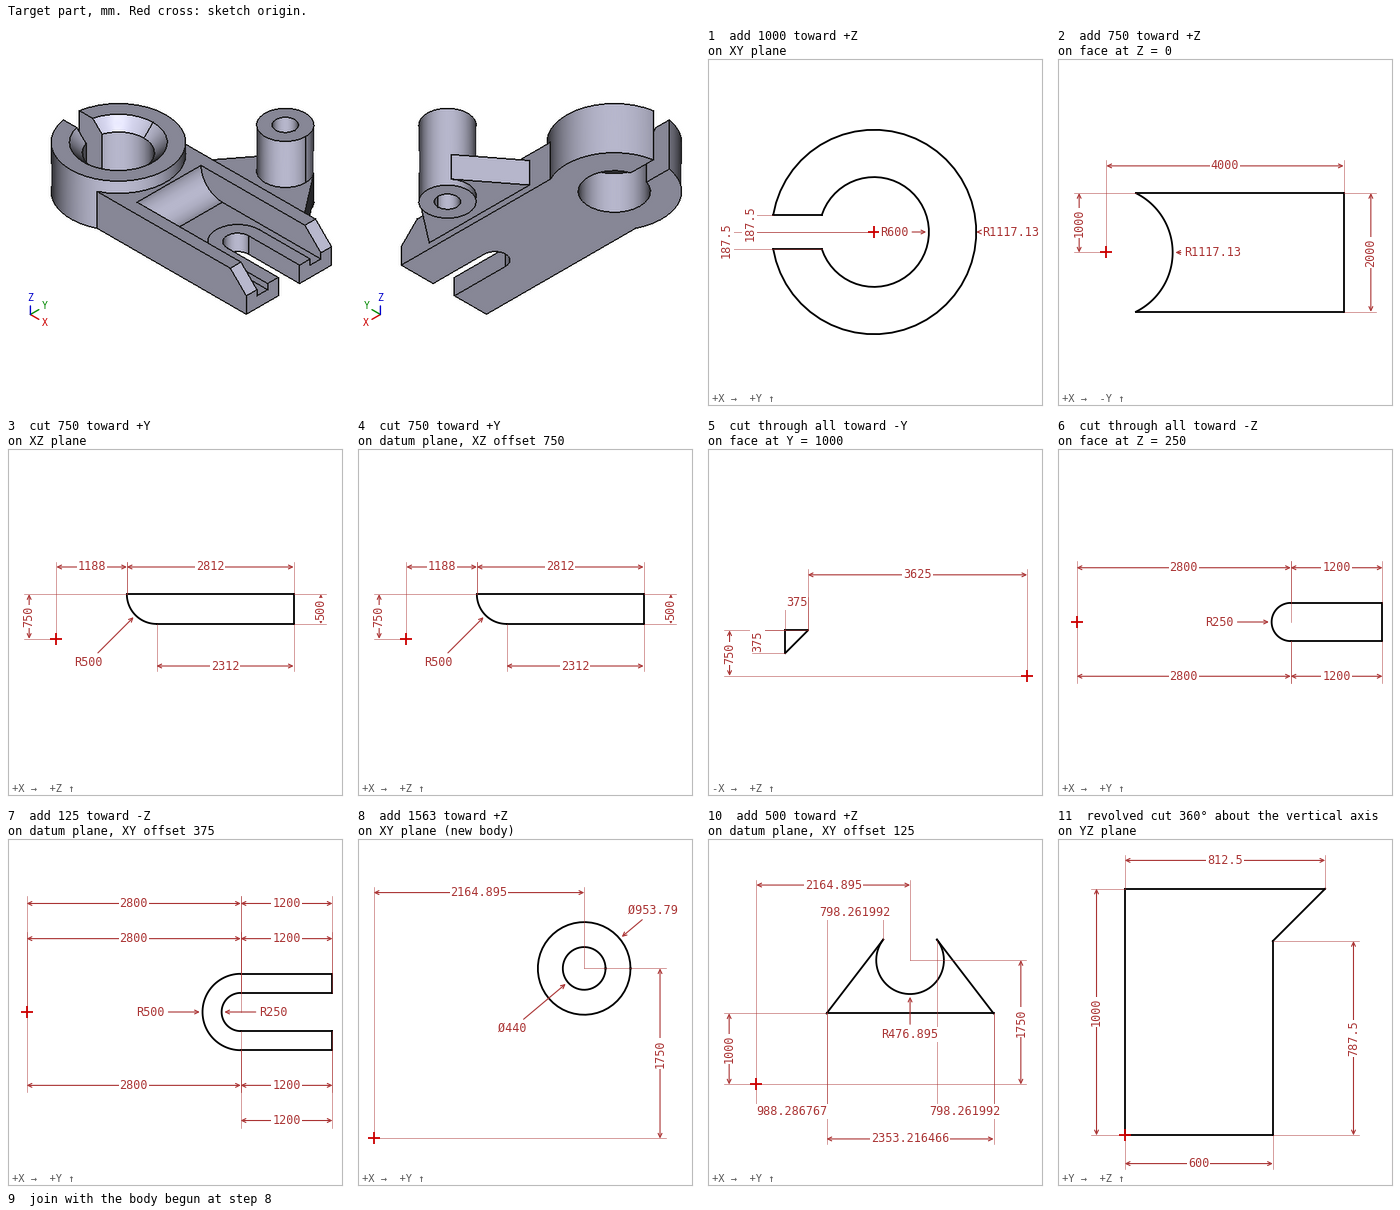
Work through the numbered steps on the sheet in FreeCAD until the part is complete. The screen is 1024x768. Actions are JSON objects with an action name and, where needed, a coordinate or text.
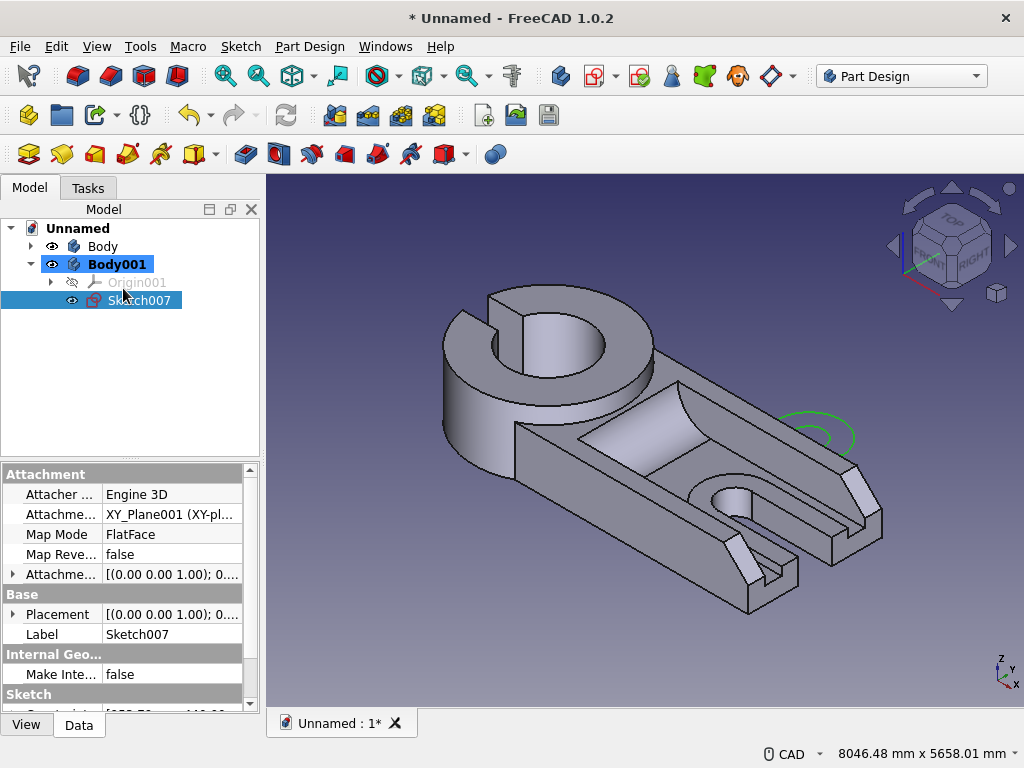
{"action": "left_click", "coordinate": [29, 154]}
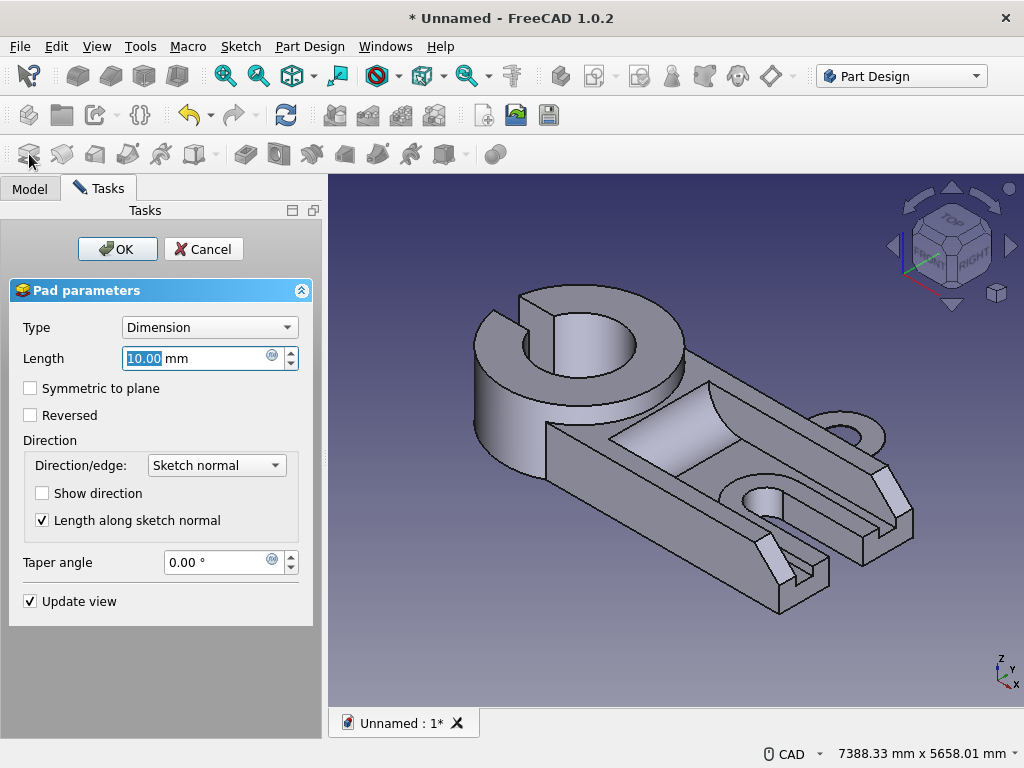
{"action": "type", "text": "1563"}
{"action": "key", "text": "Tab"}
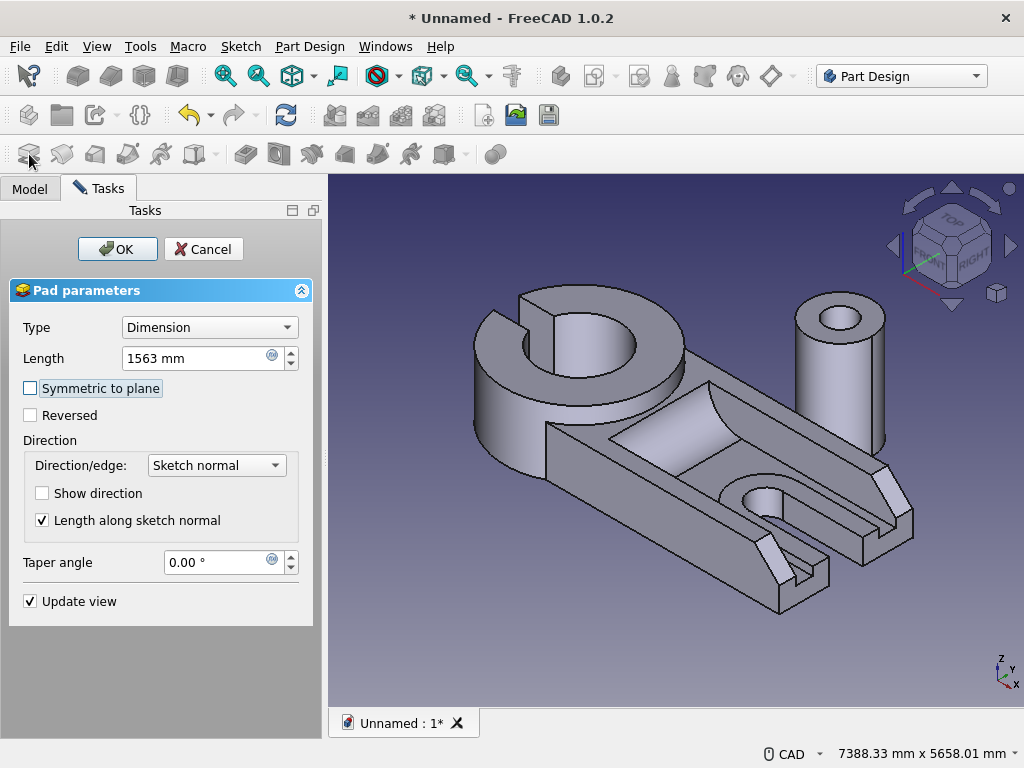
{"action": "left_click", "coordinate": [118, 249]}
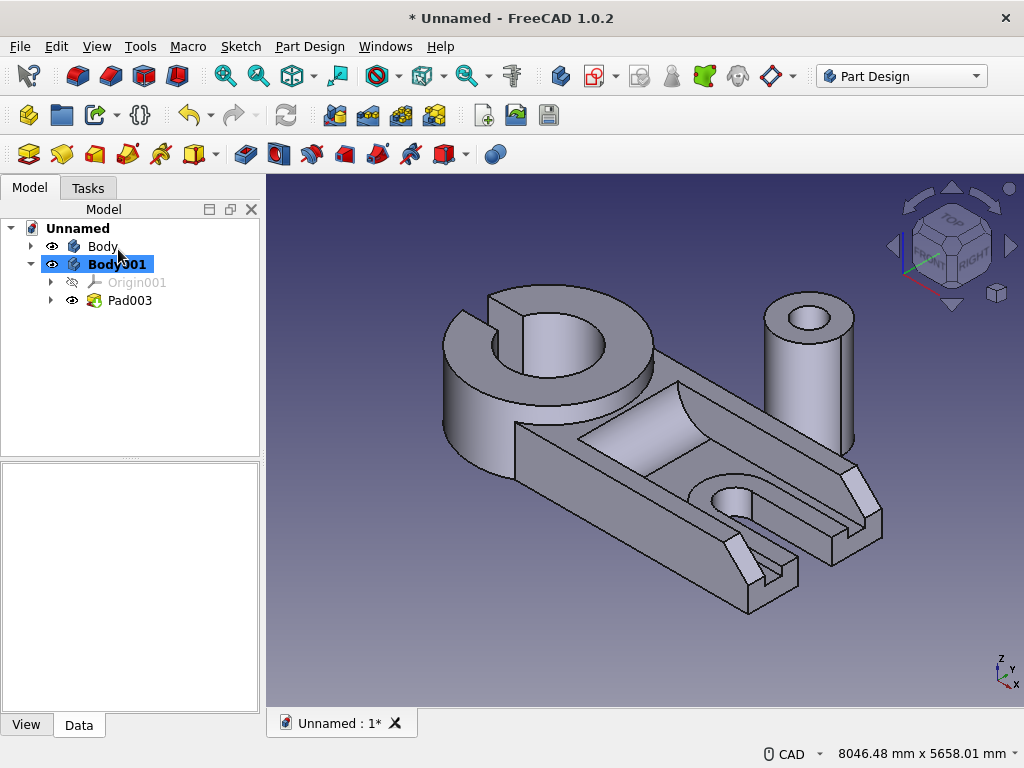
{"action": "key", "text": "v f"}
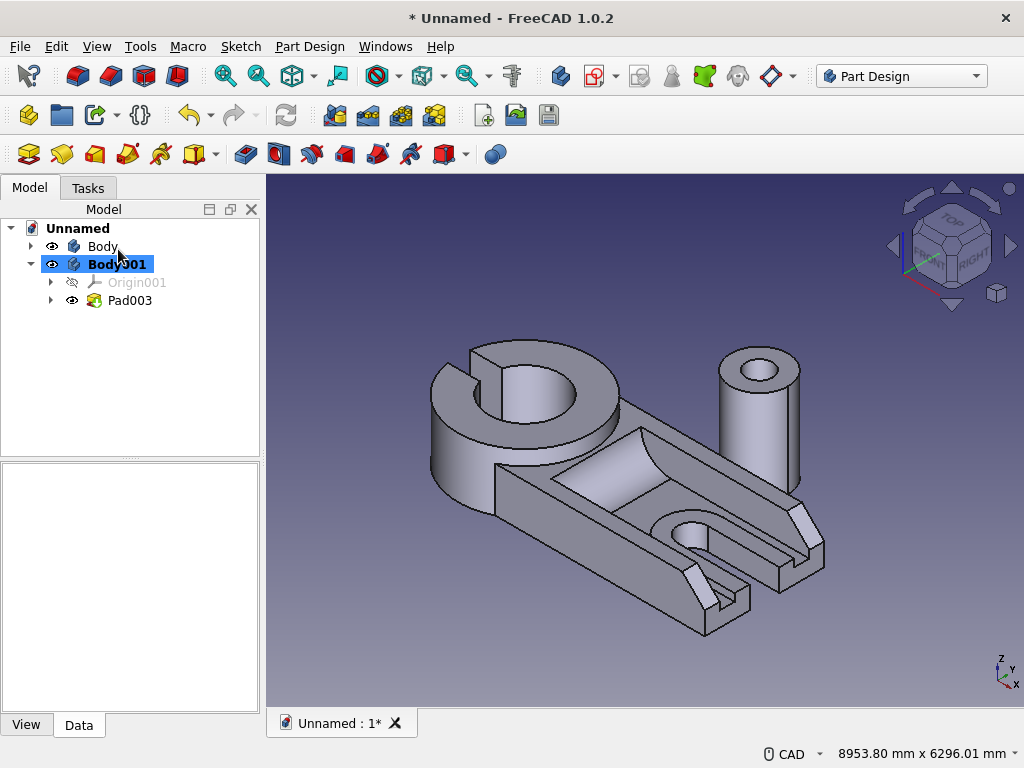
{"action": "double_click", "coordinate": [97, 246]}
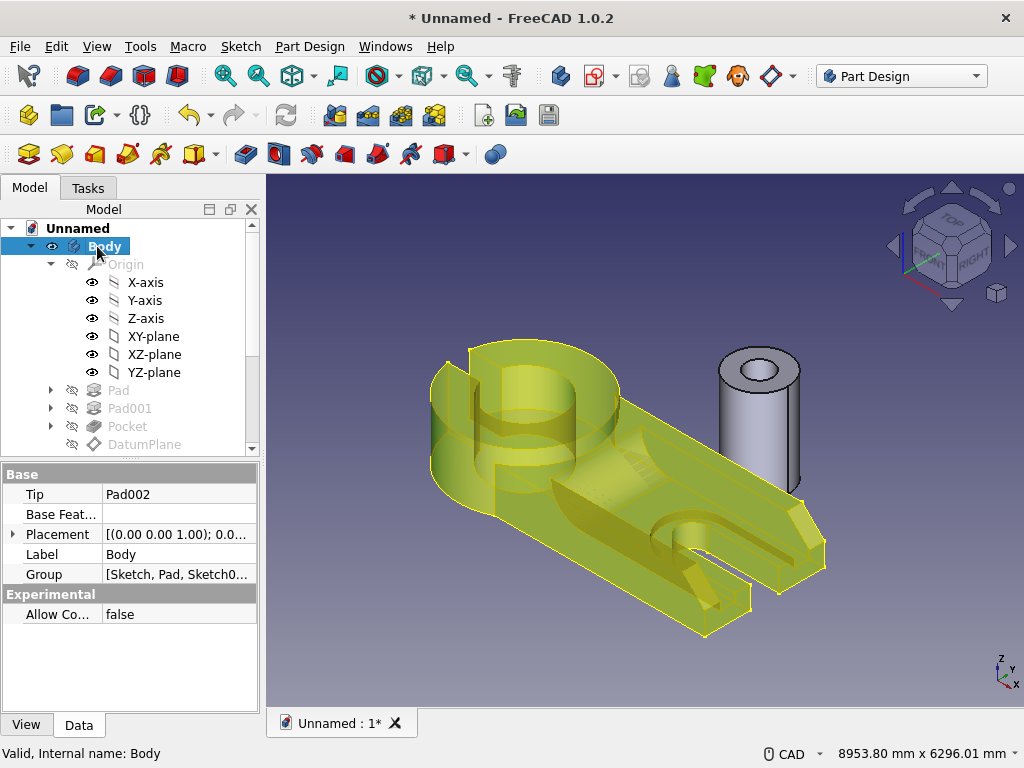
{"action": "left_click", "coordinate": [97, 246]}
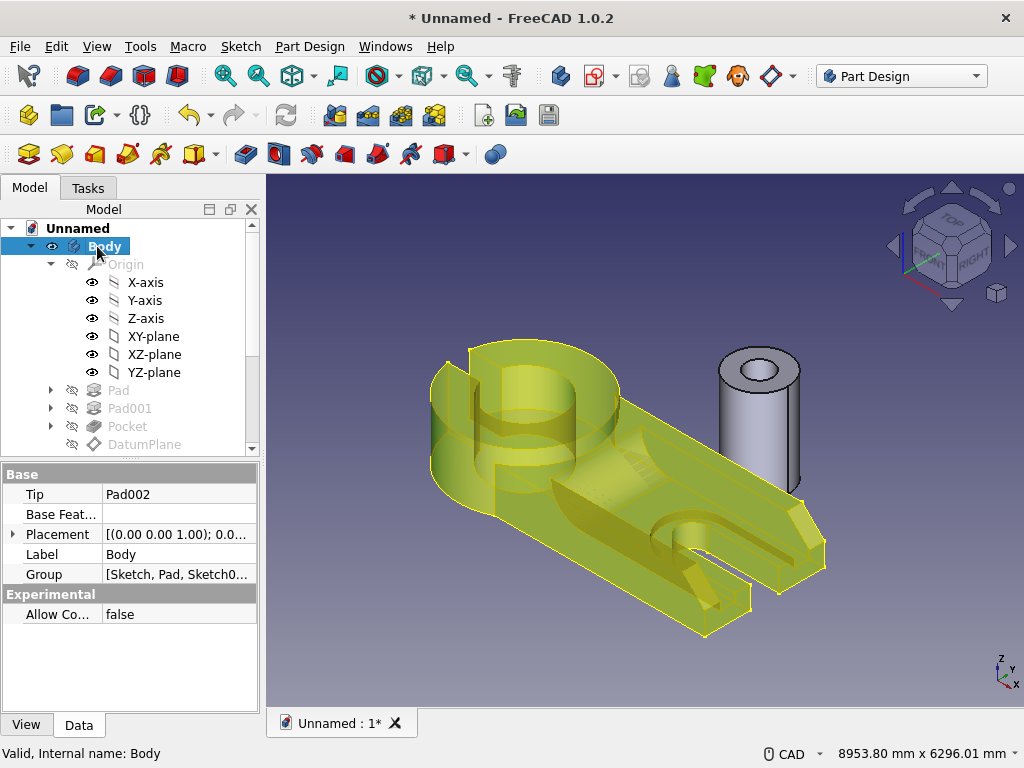
{"action": "left_click", "coordinate": [148, 614]}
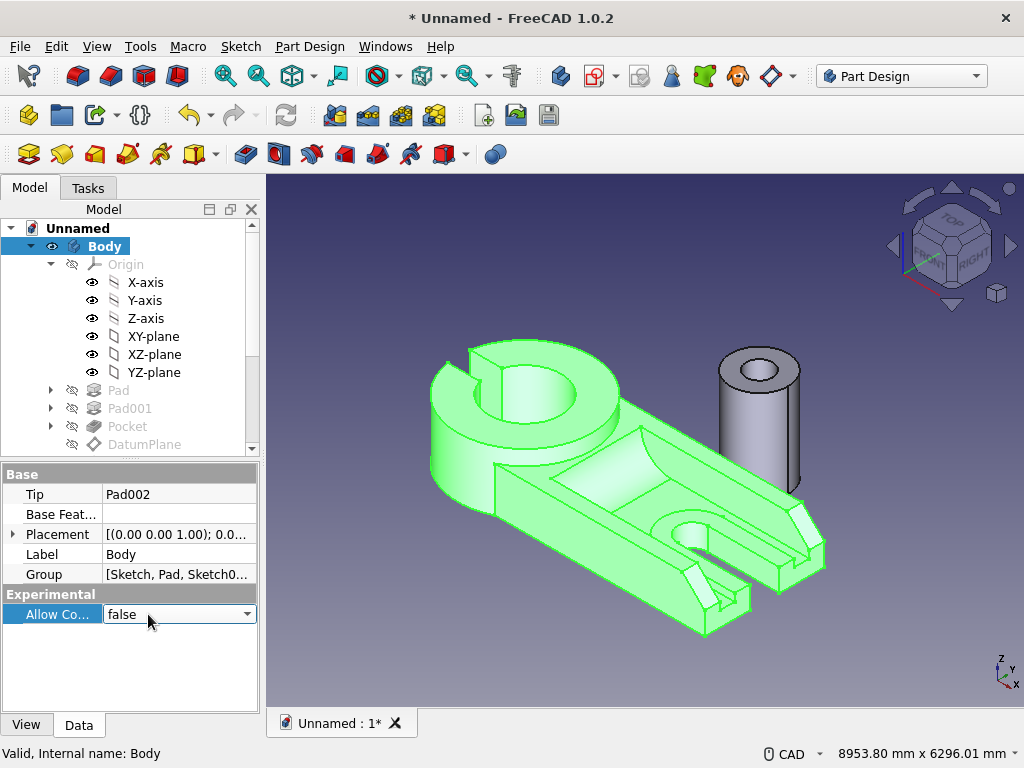
{"action": "left_click", "coordinate": [148, 614]}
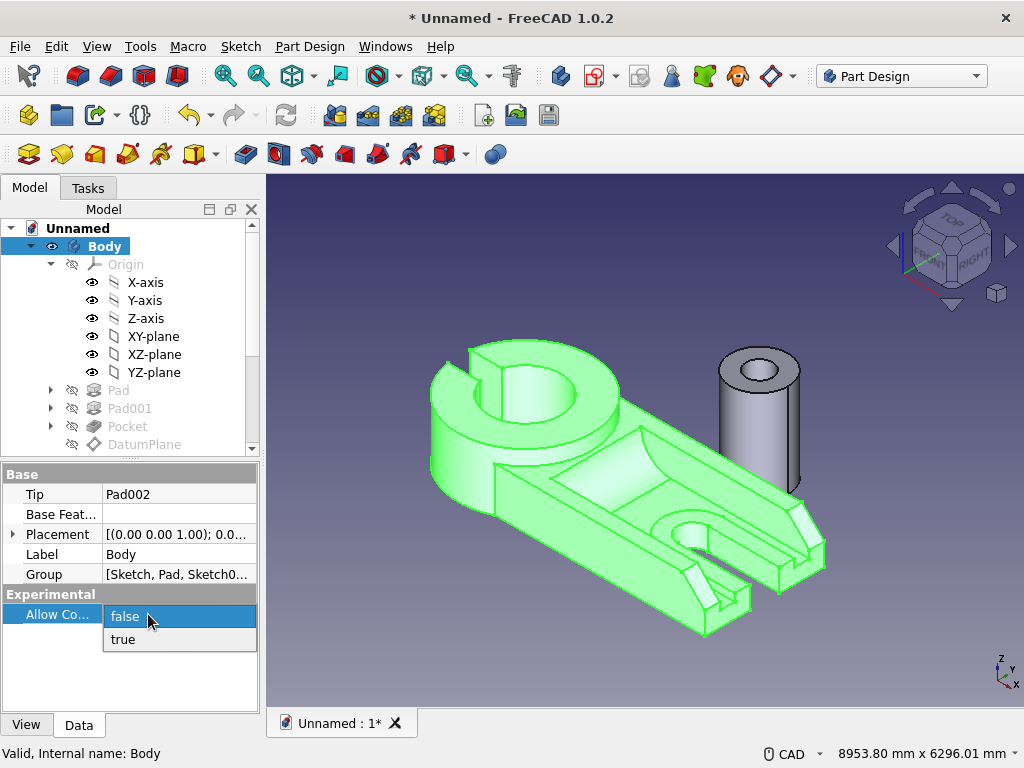
{"action": "left_click", "coordinate": [178, 640]}
{"action": "key", "text": "Return"}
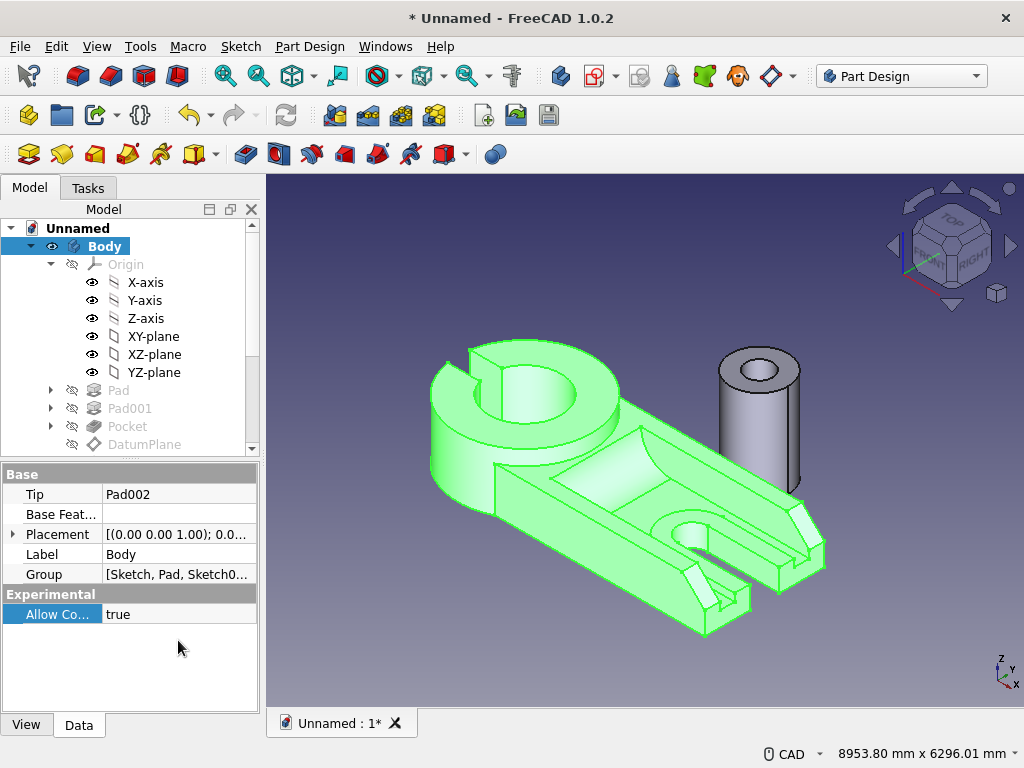
{"action": "scroll", "coordinate": [101, 332], "scroll_direction": "down", "scroll_amount": 3}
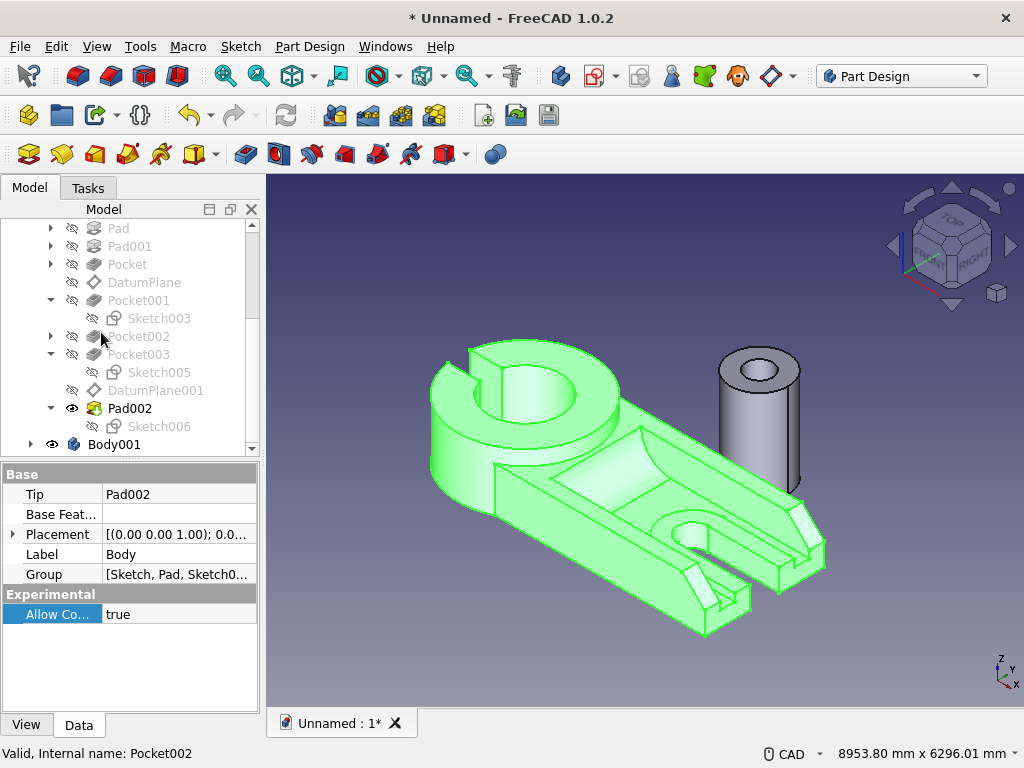
{"action": "left_click", "coordinate": [97, 444]}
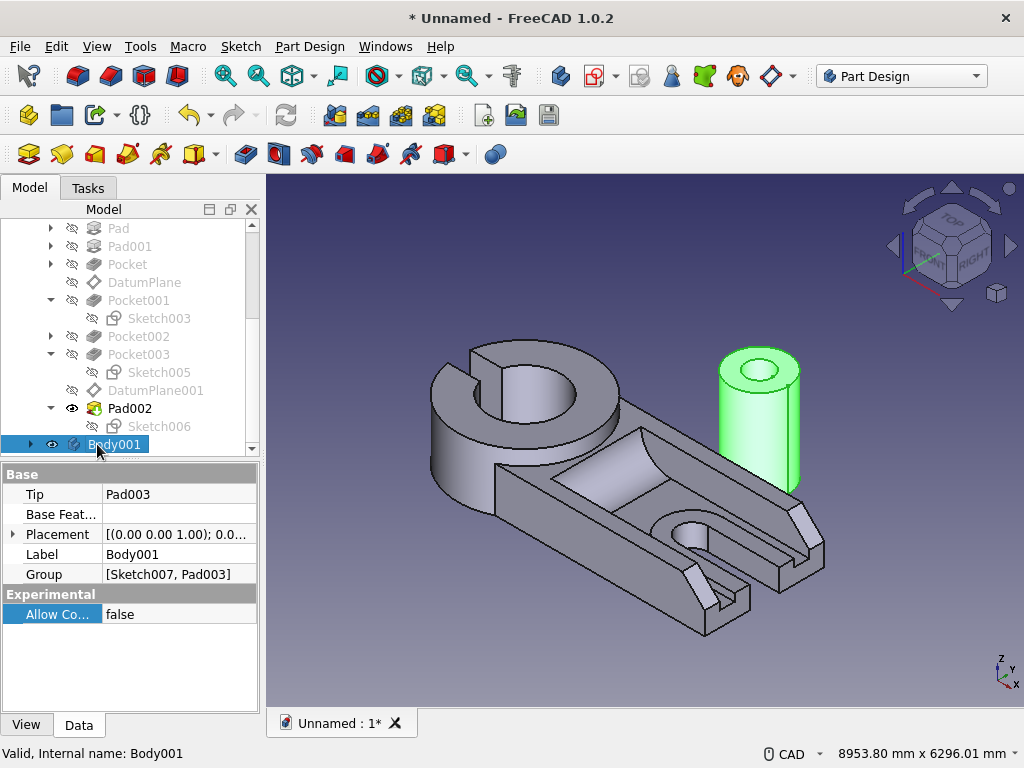
{"action": "left_click", "coordinate": [496, 154]}